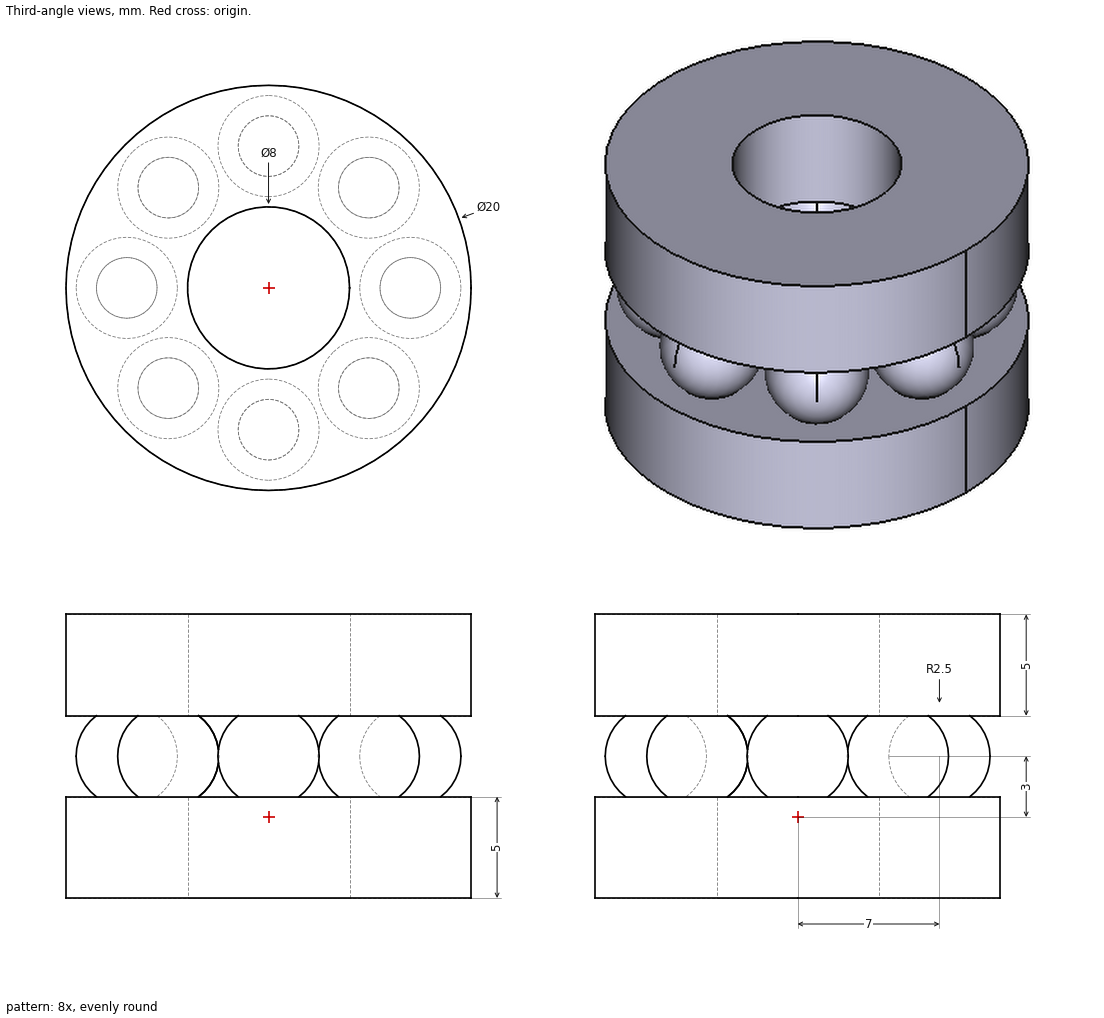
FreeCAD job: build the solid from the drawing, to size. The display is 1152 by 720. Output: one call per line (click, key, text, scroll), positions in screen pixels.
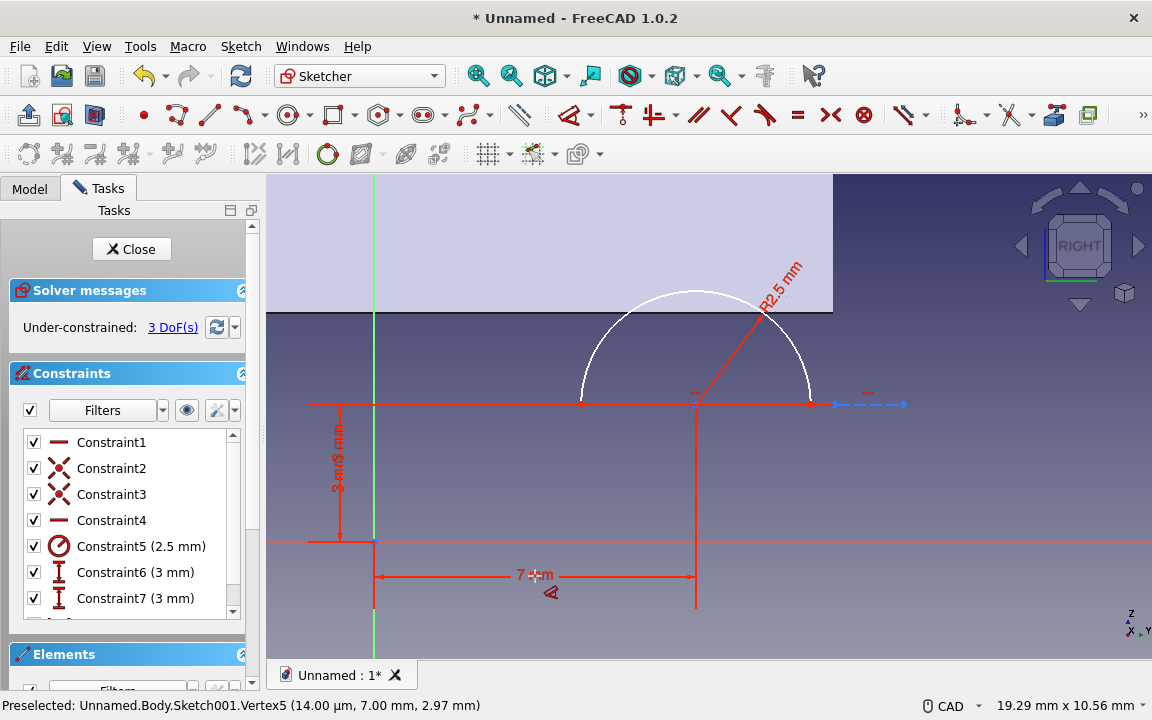
click(696, 406)
click(340, 506)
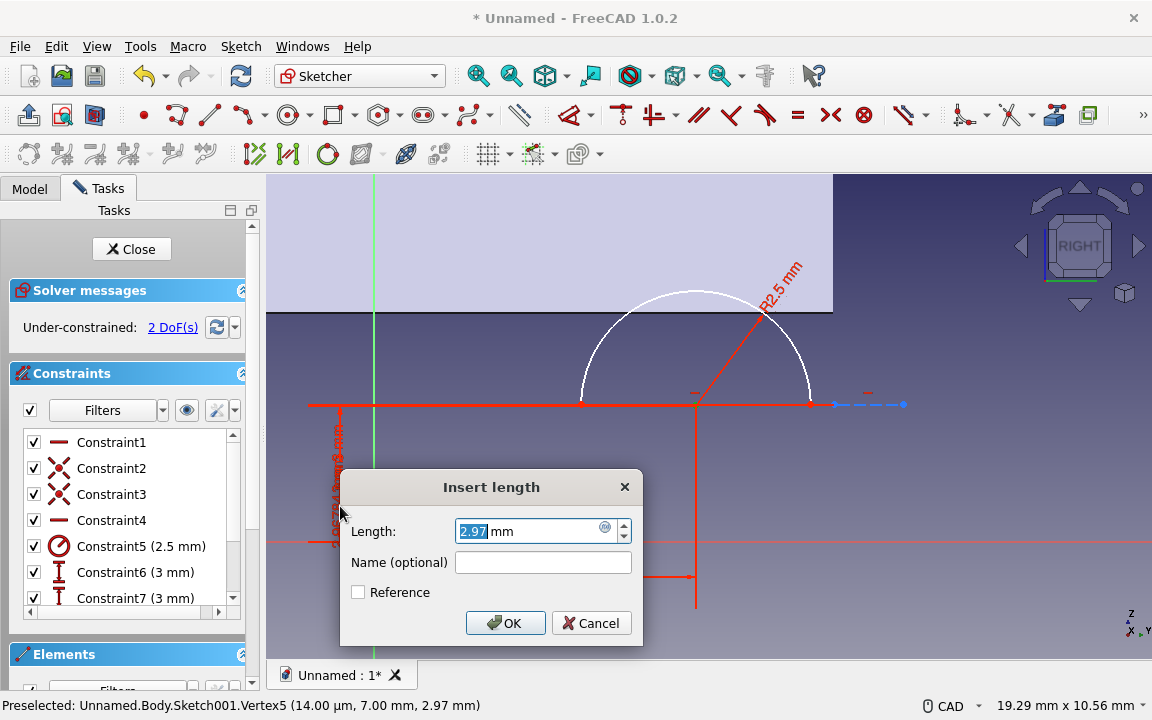
text(3)
key(Return)
key(Escape)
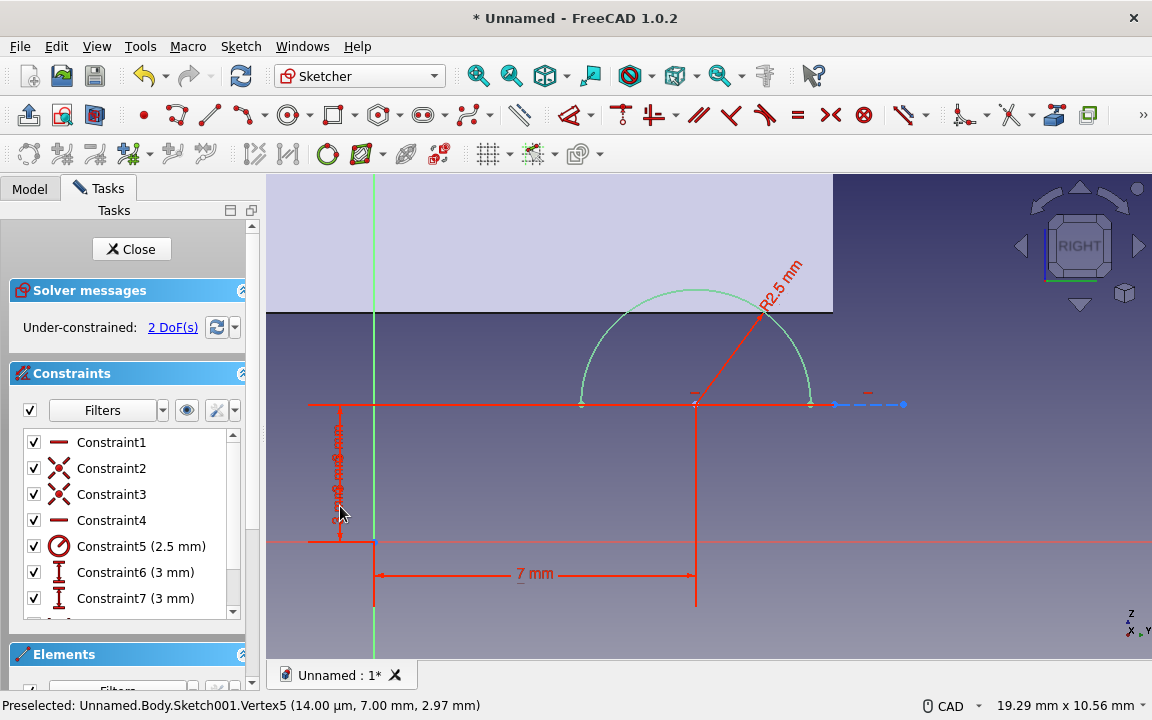
click(132, 249)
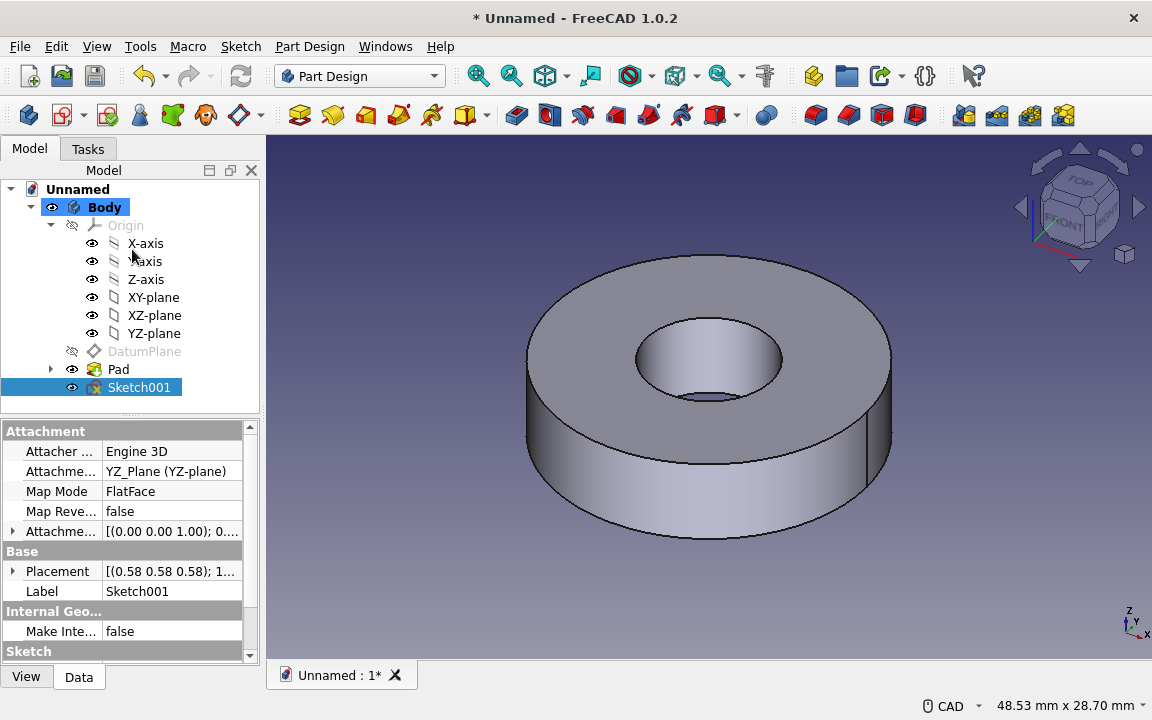
click(333, 116)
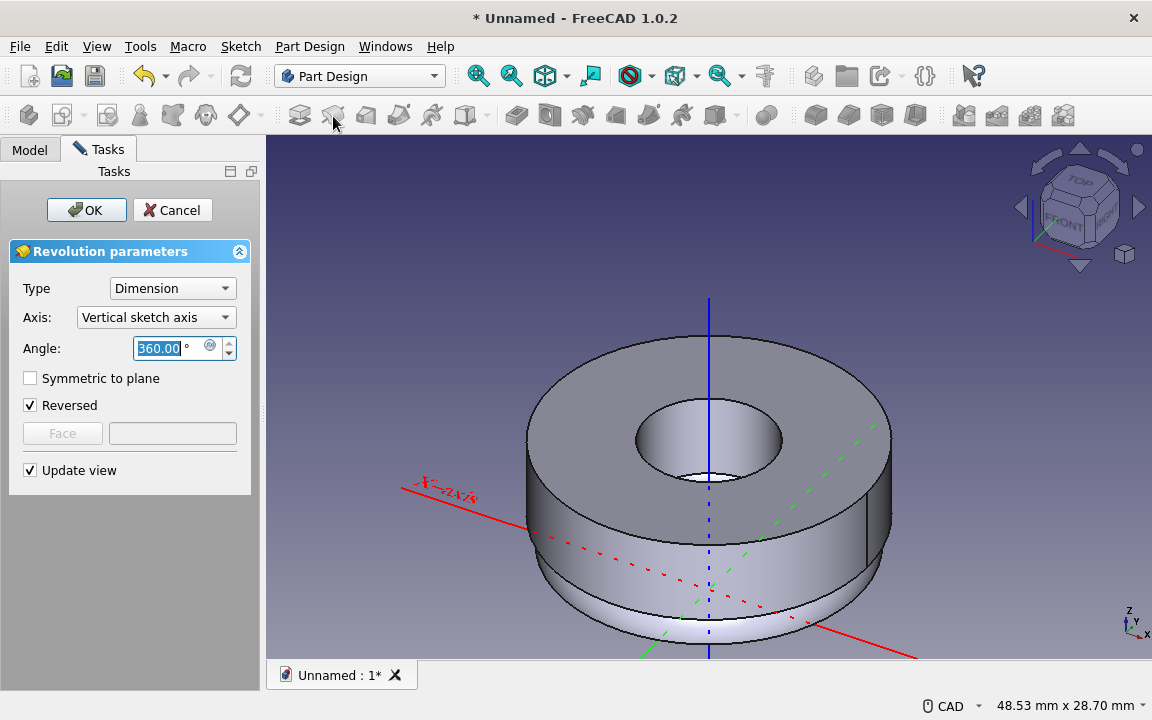
click(157, 318)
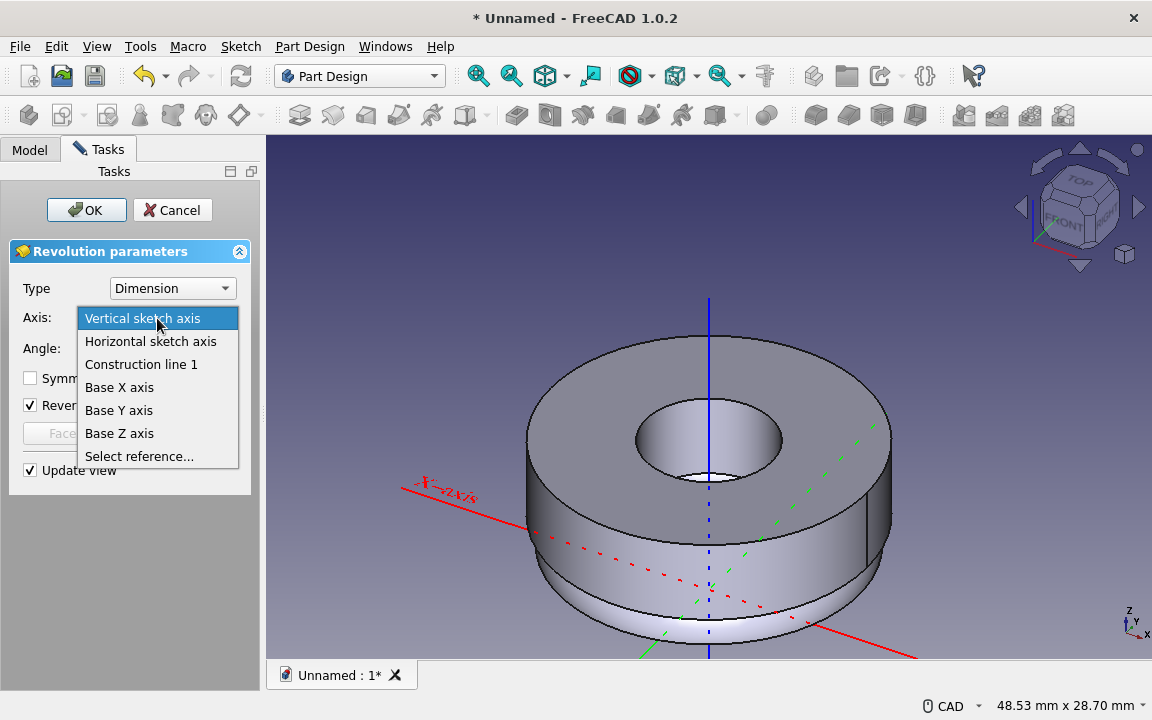
click(156, 364)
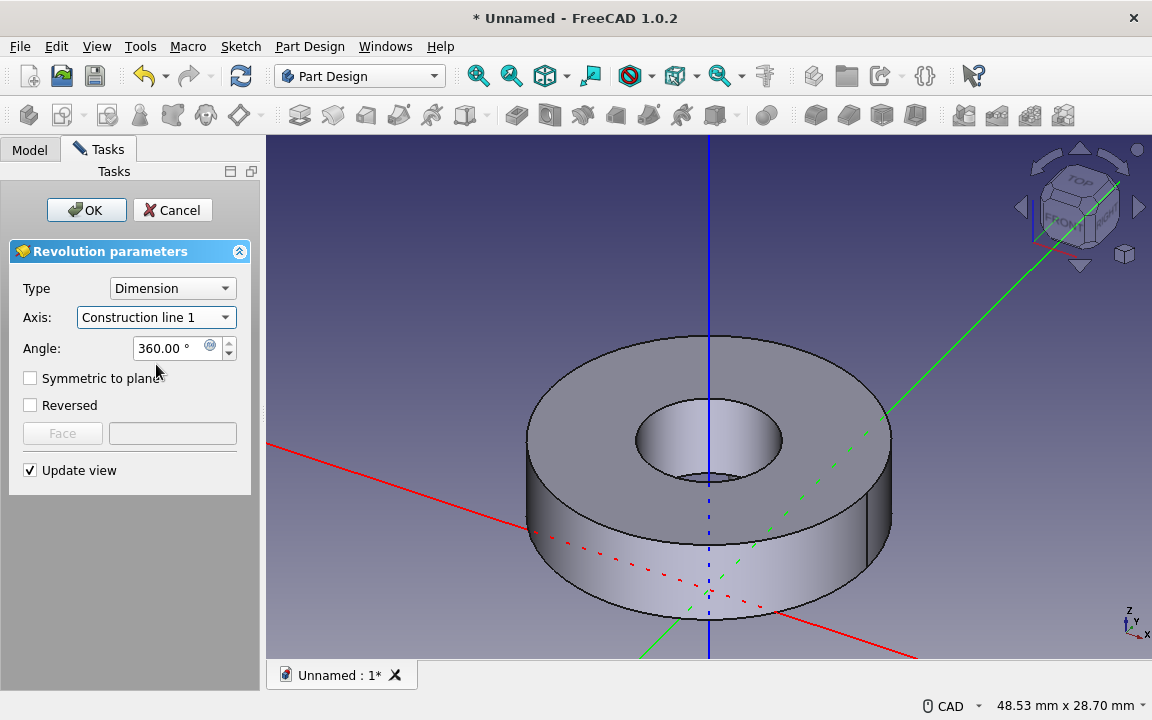
click(87, 210)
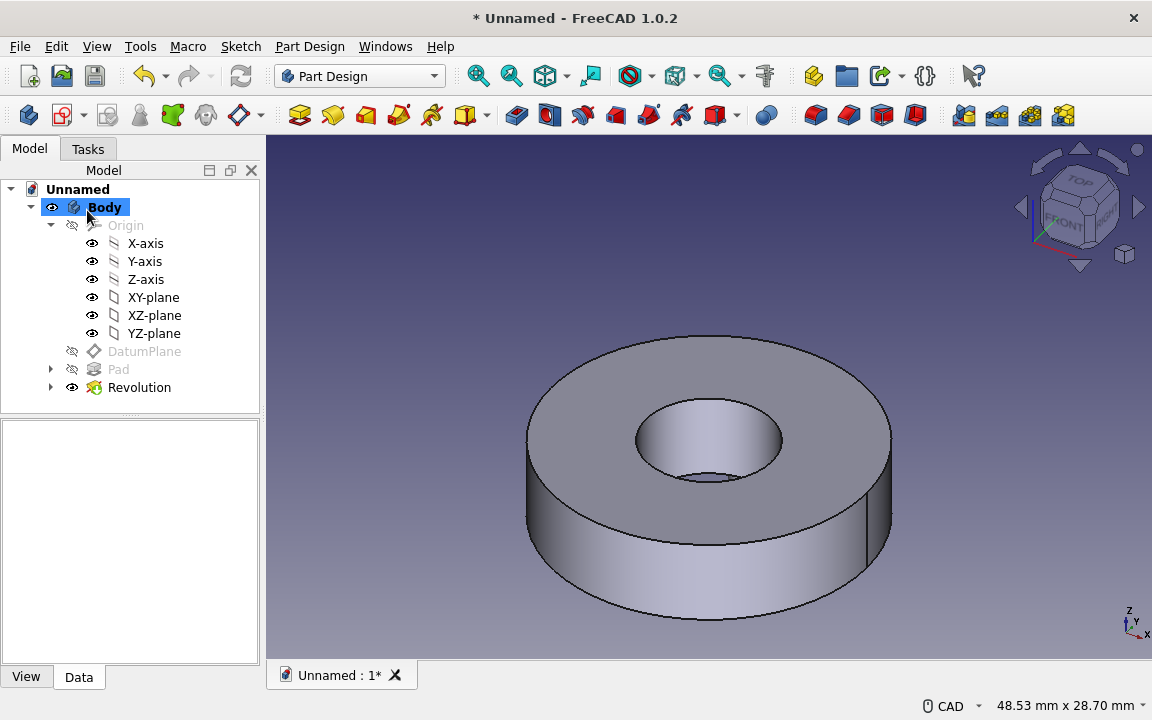
click(479, 76)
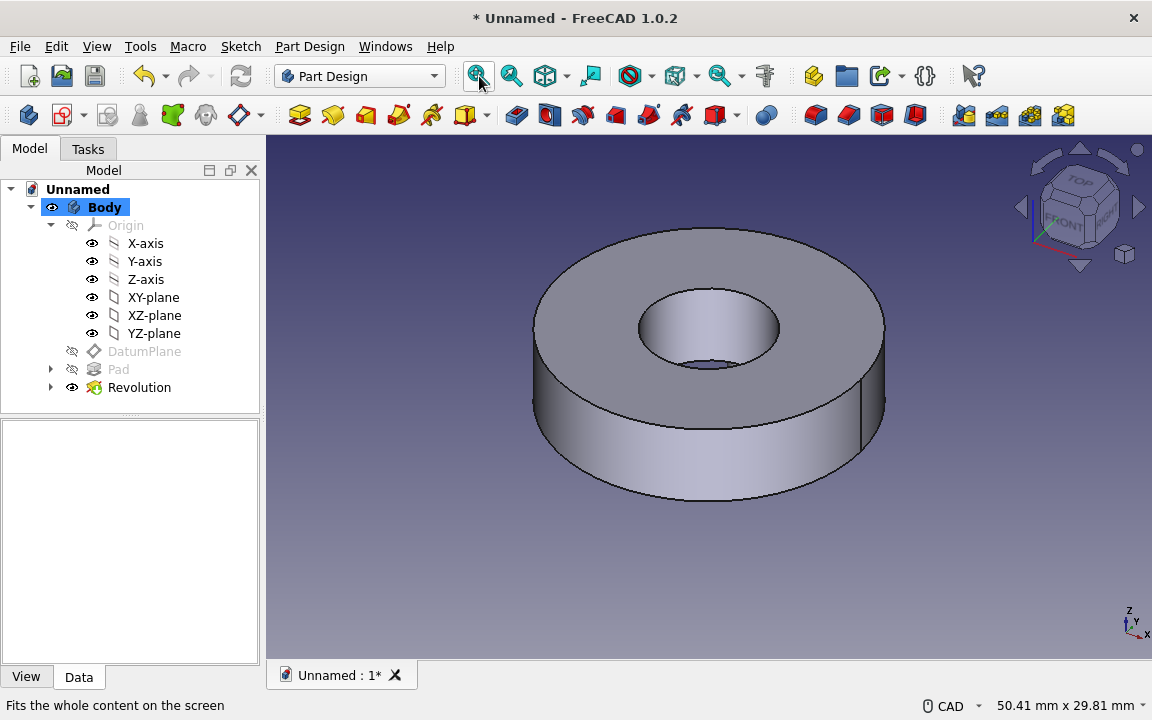
click(117, 387)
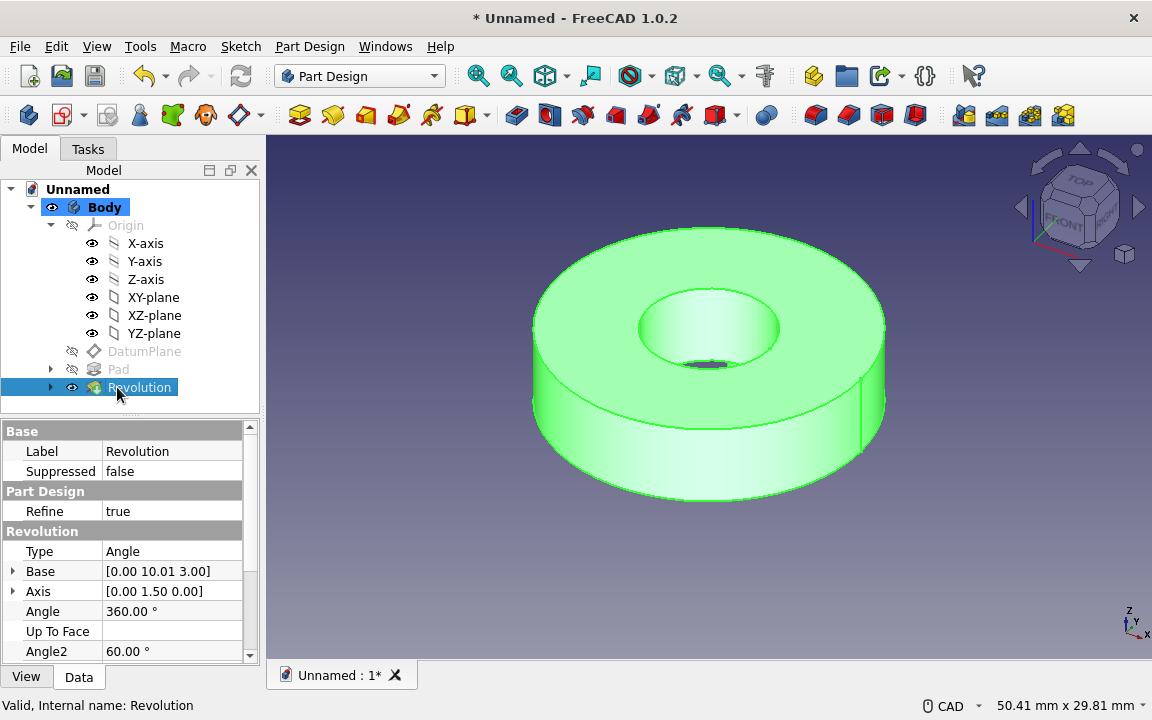
click(1030, 116)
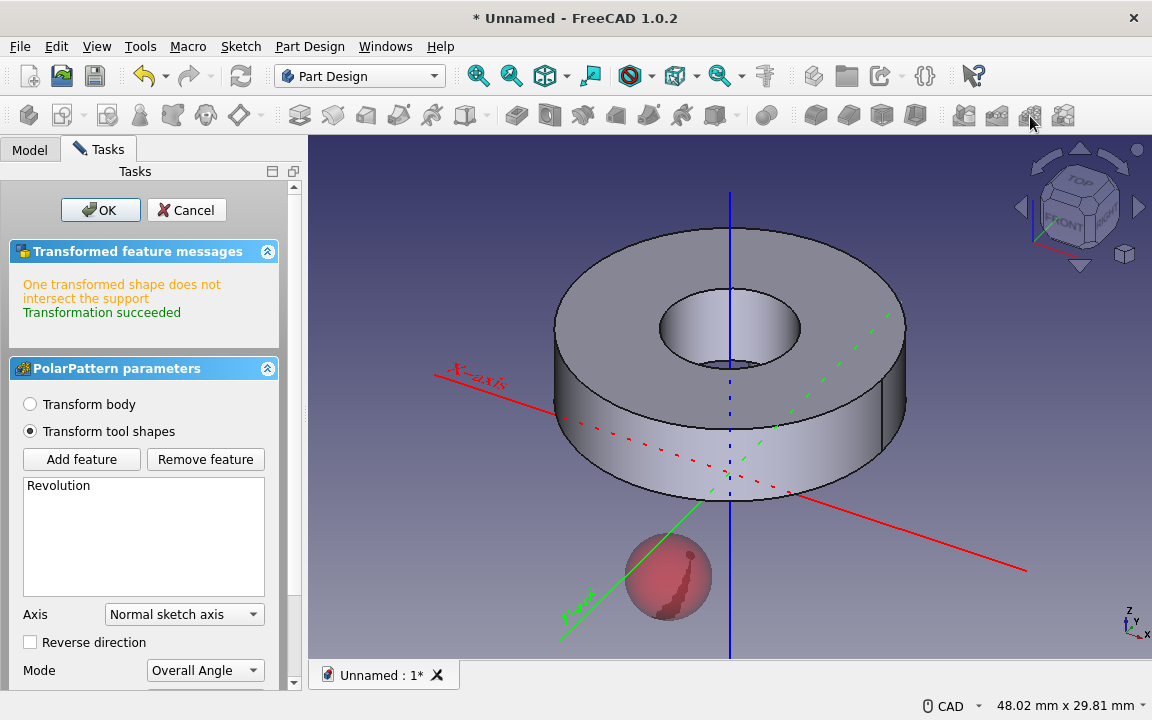
click(185, 614)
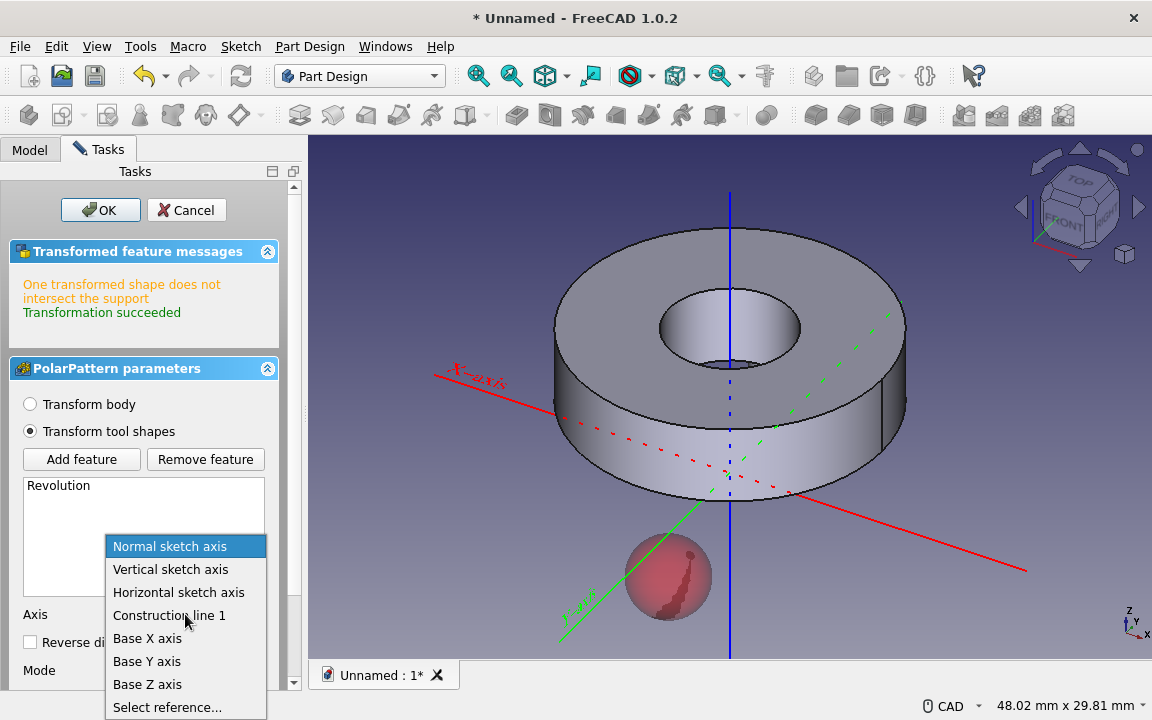
click(184, 684)